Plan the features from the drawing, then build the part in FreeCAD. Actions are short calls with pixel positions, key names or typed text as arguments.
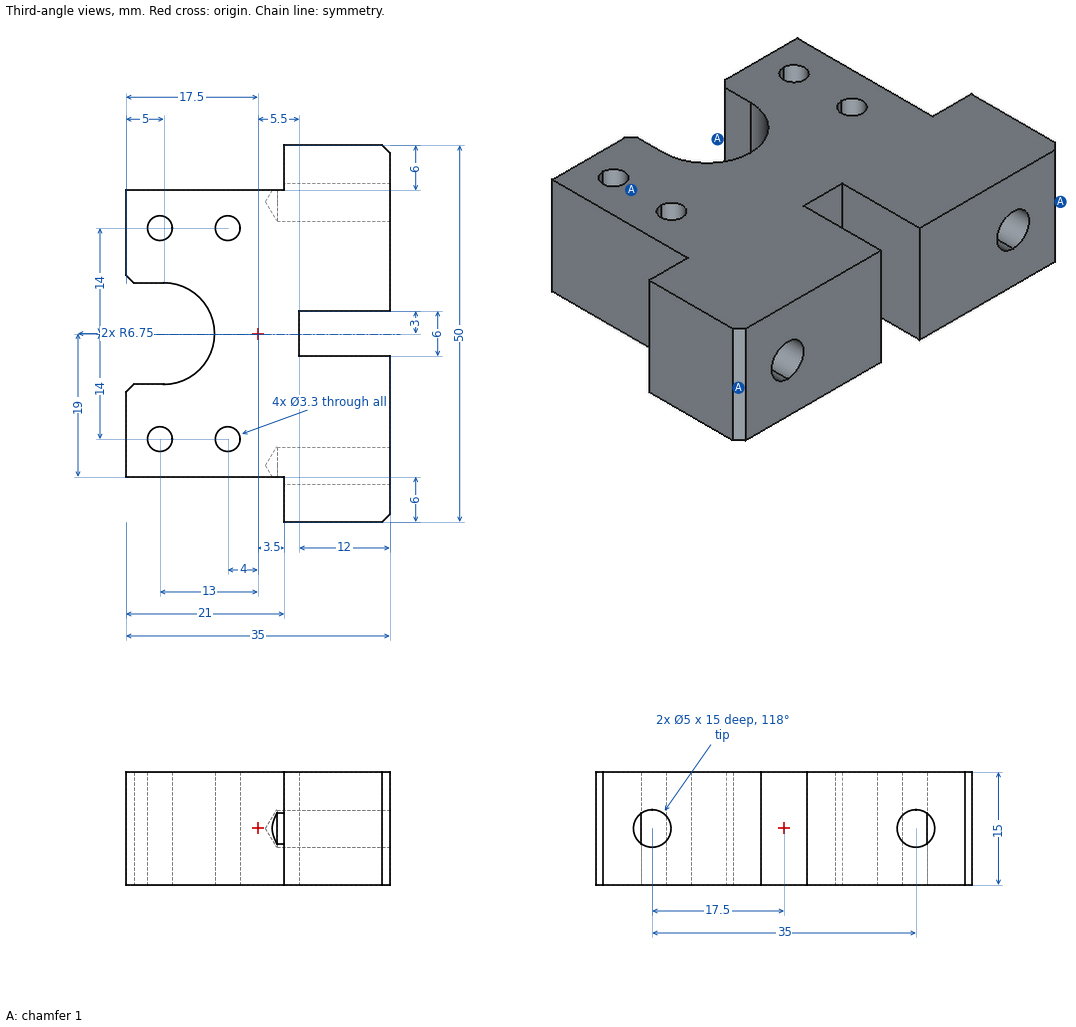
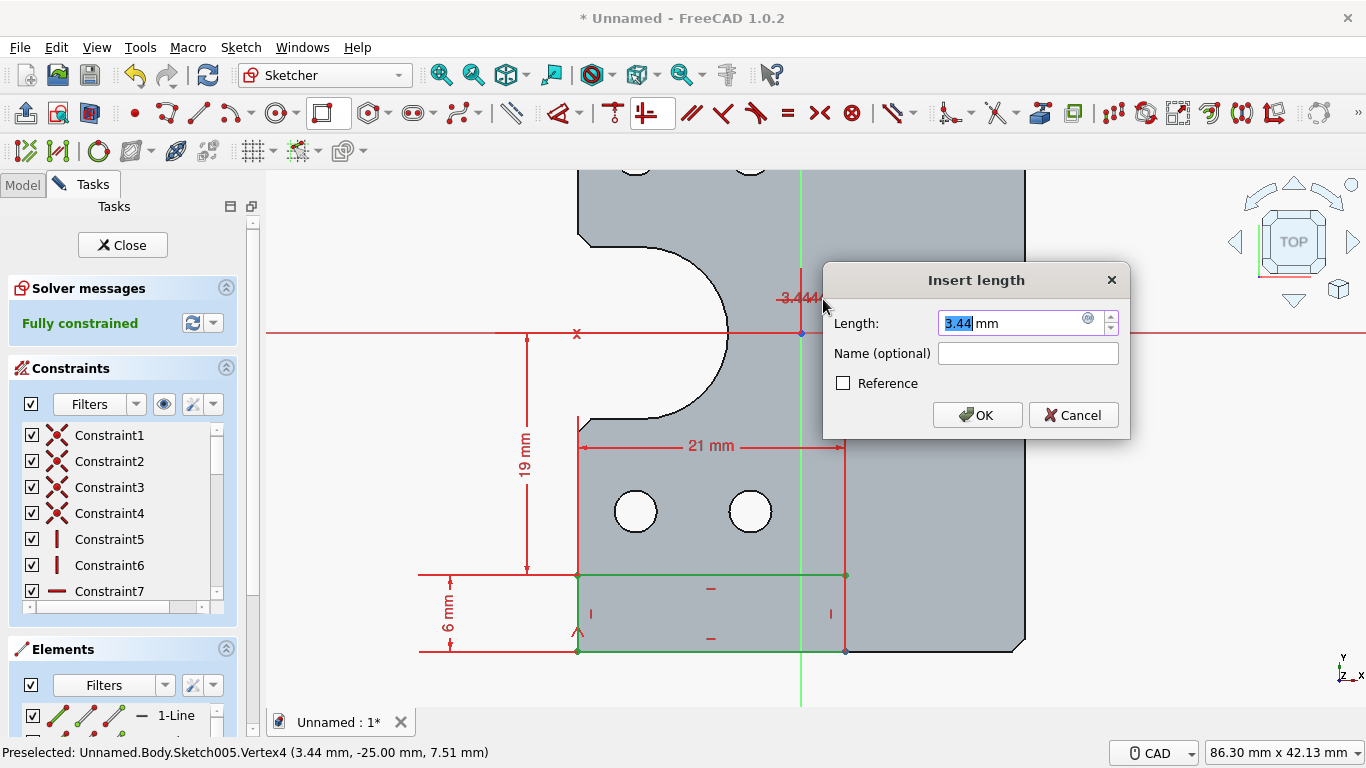
text(3.5)
key(Return)
key(Escape)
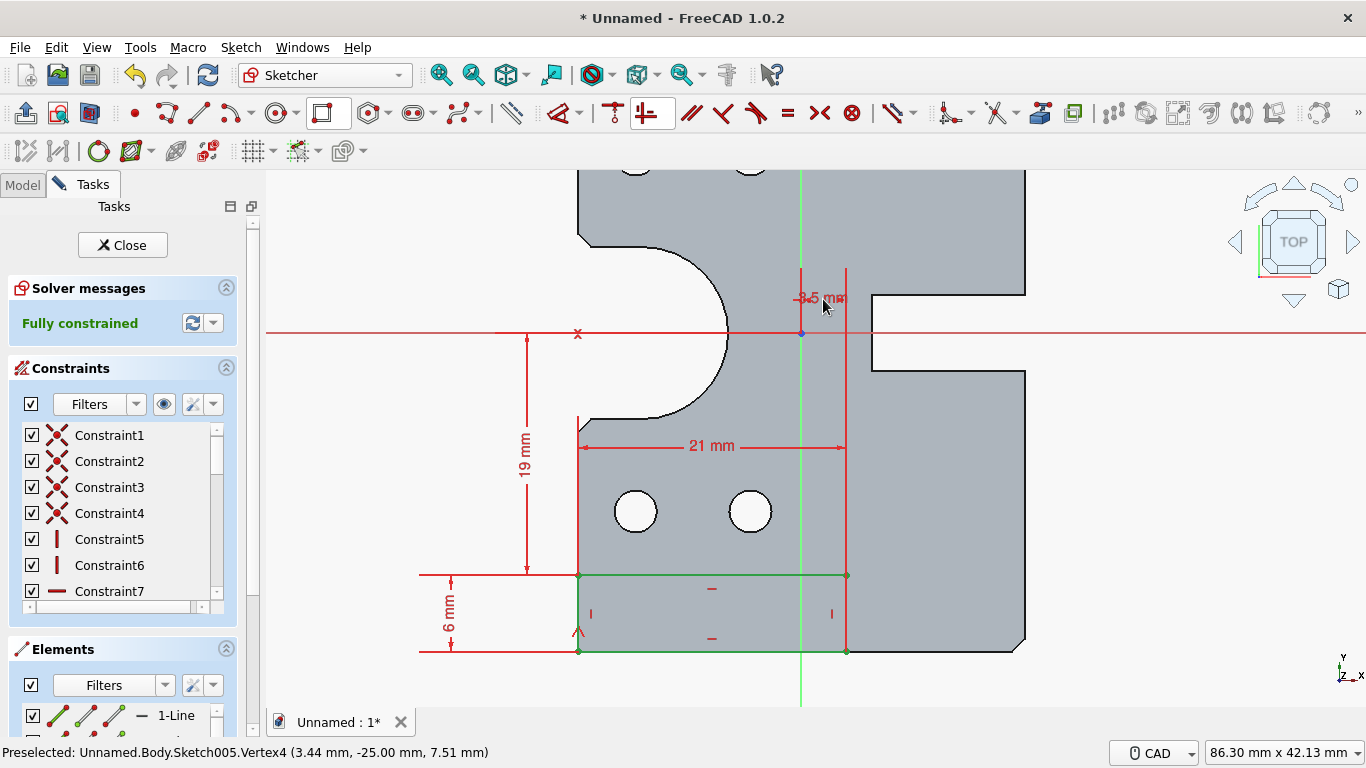
click(123, 245)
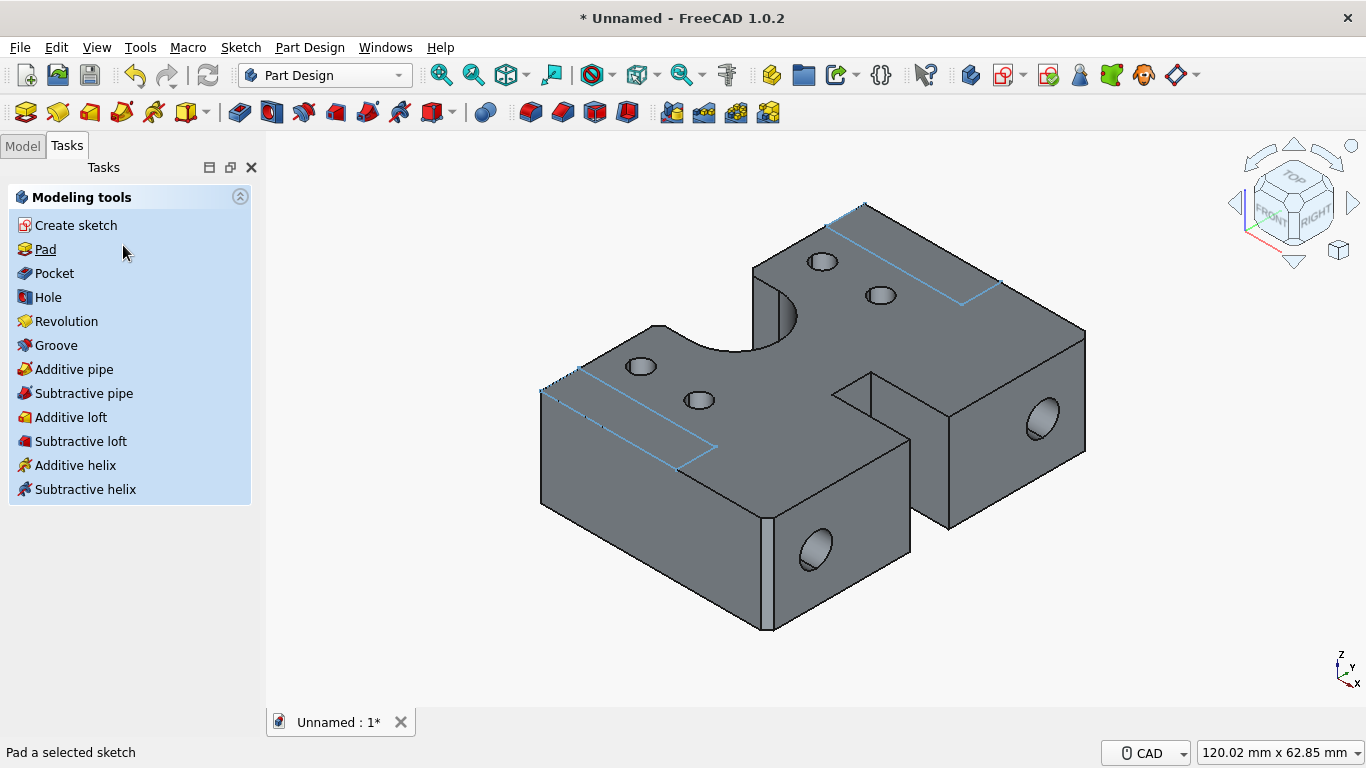
click(240, 112)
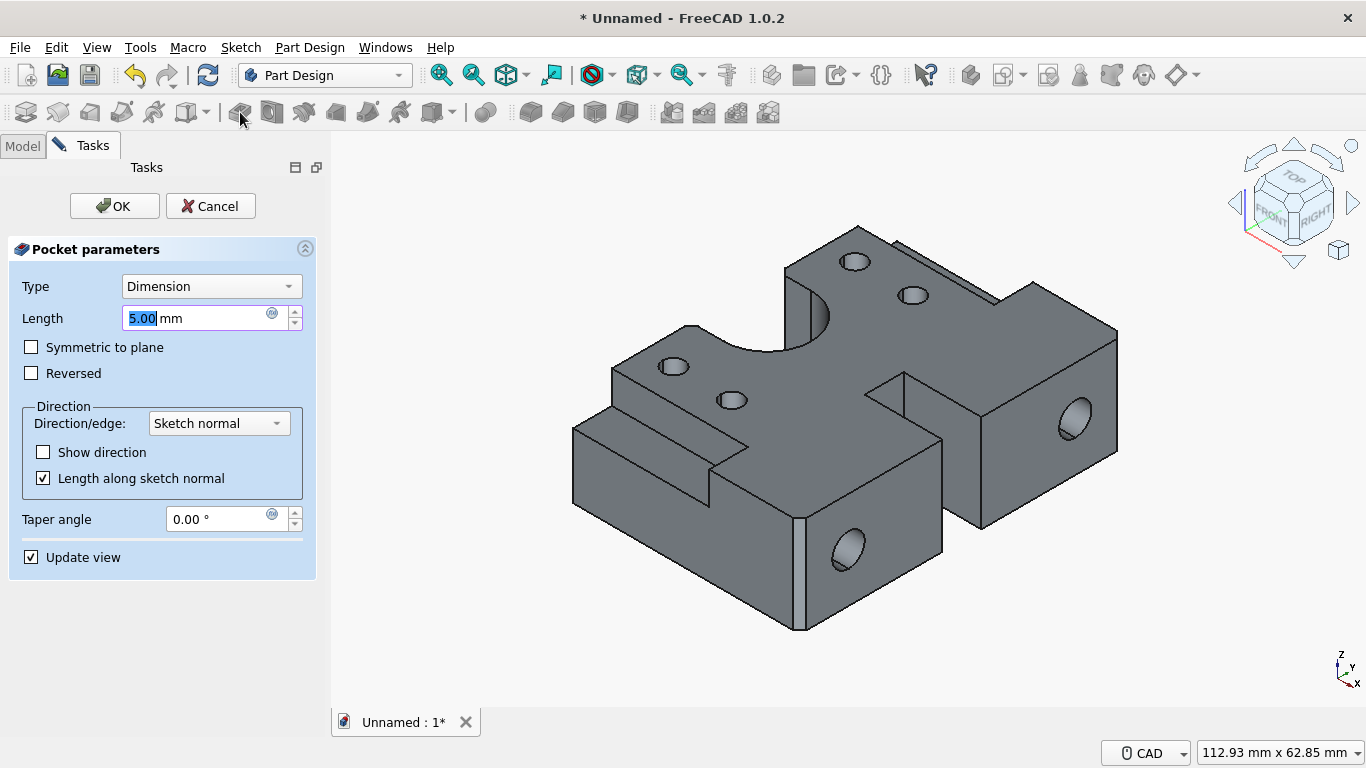
click(212, 286)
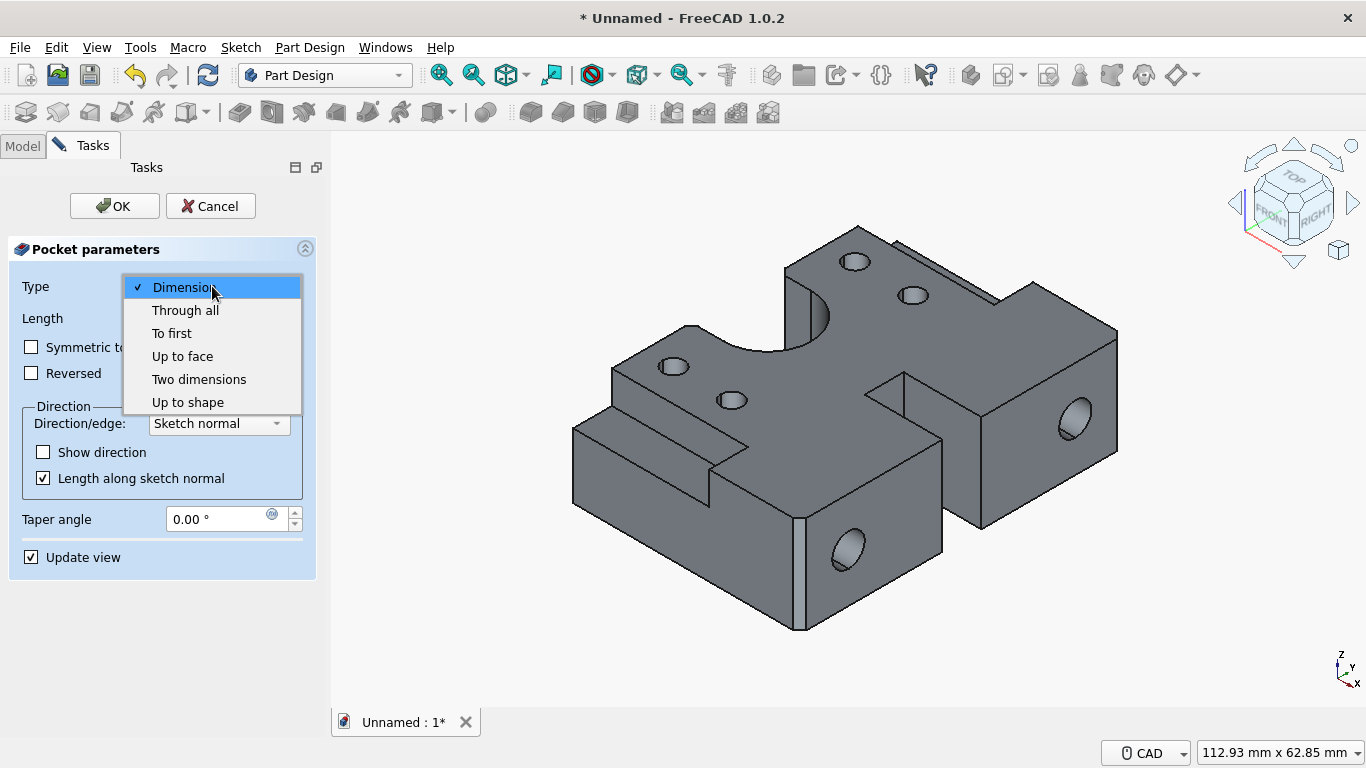
click(212, 310)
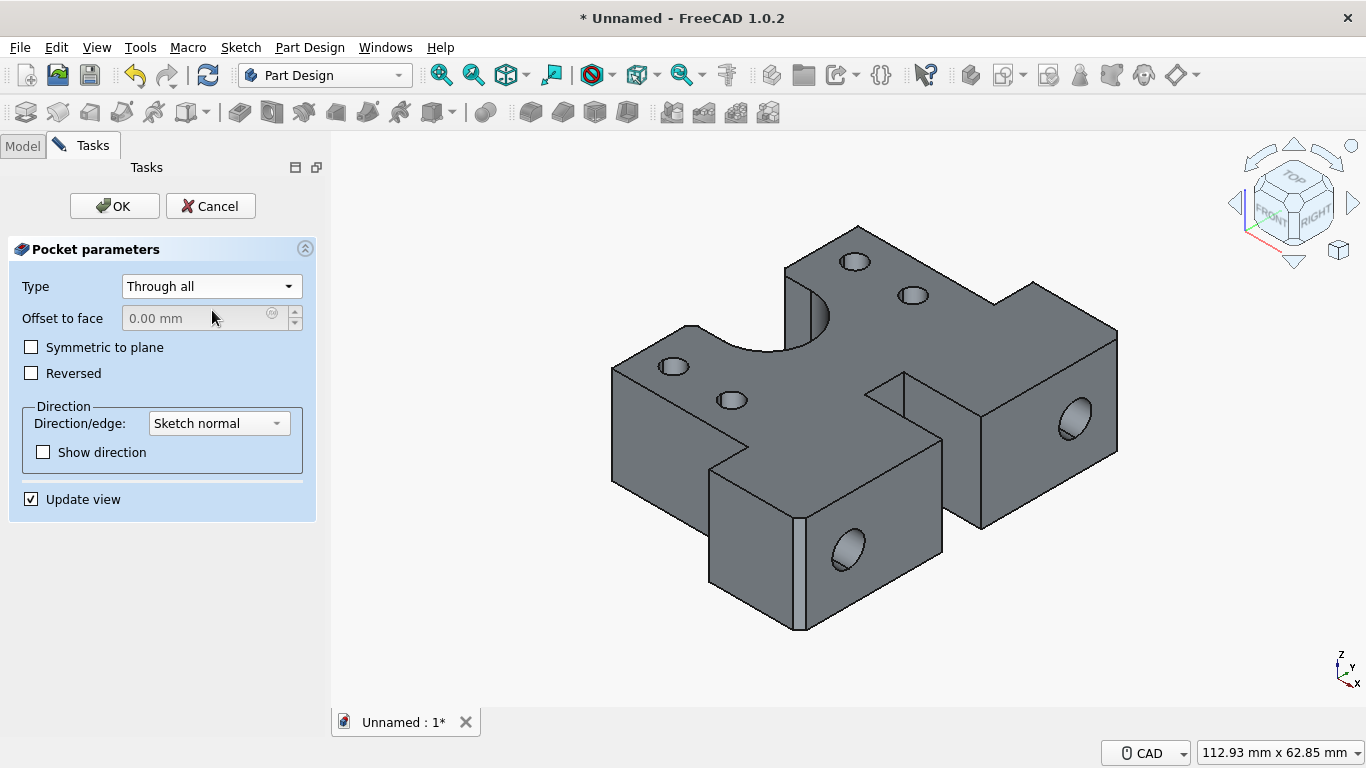
click(115, 206)